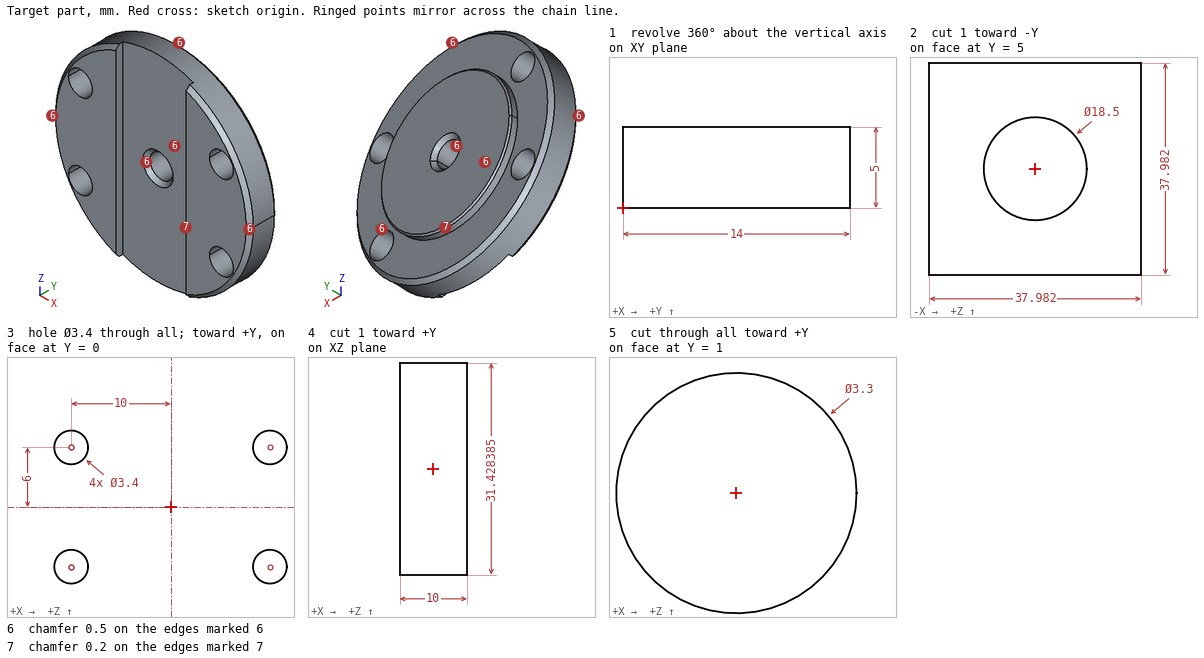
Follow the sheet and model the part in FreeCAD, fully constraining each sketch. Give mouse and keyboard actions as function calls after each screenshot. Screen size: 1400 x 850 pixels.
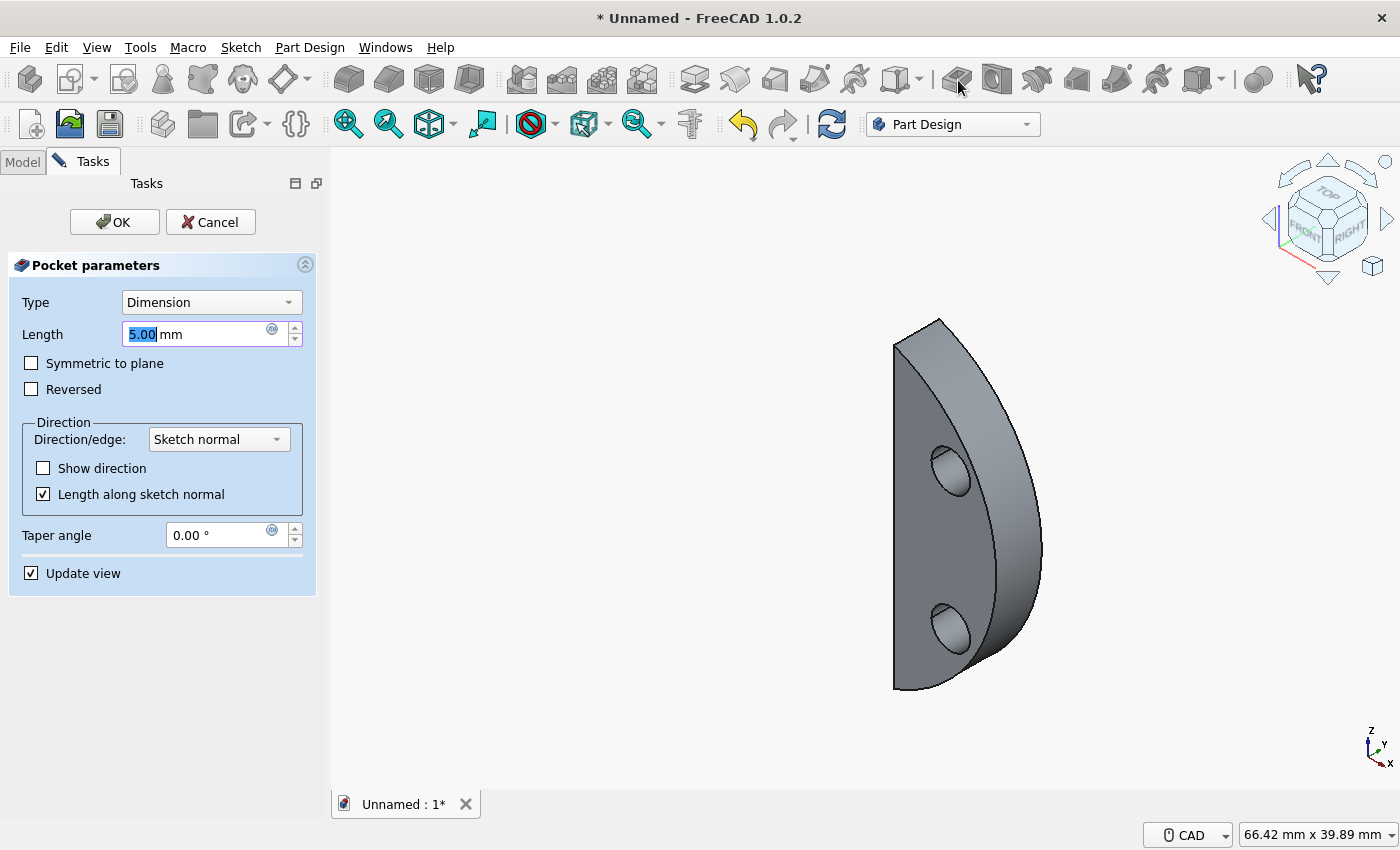
text(1)
key(Tab)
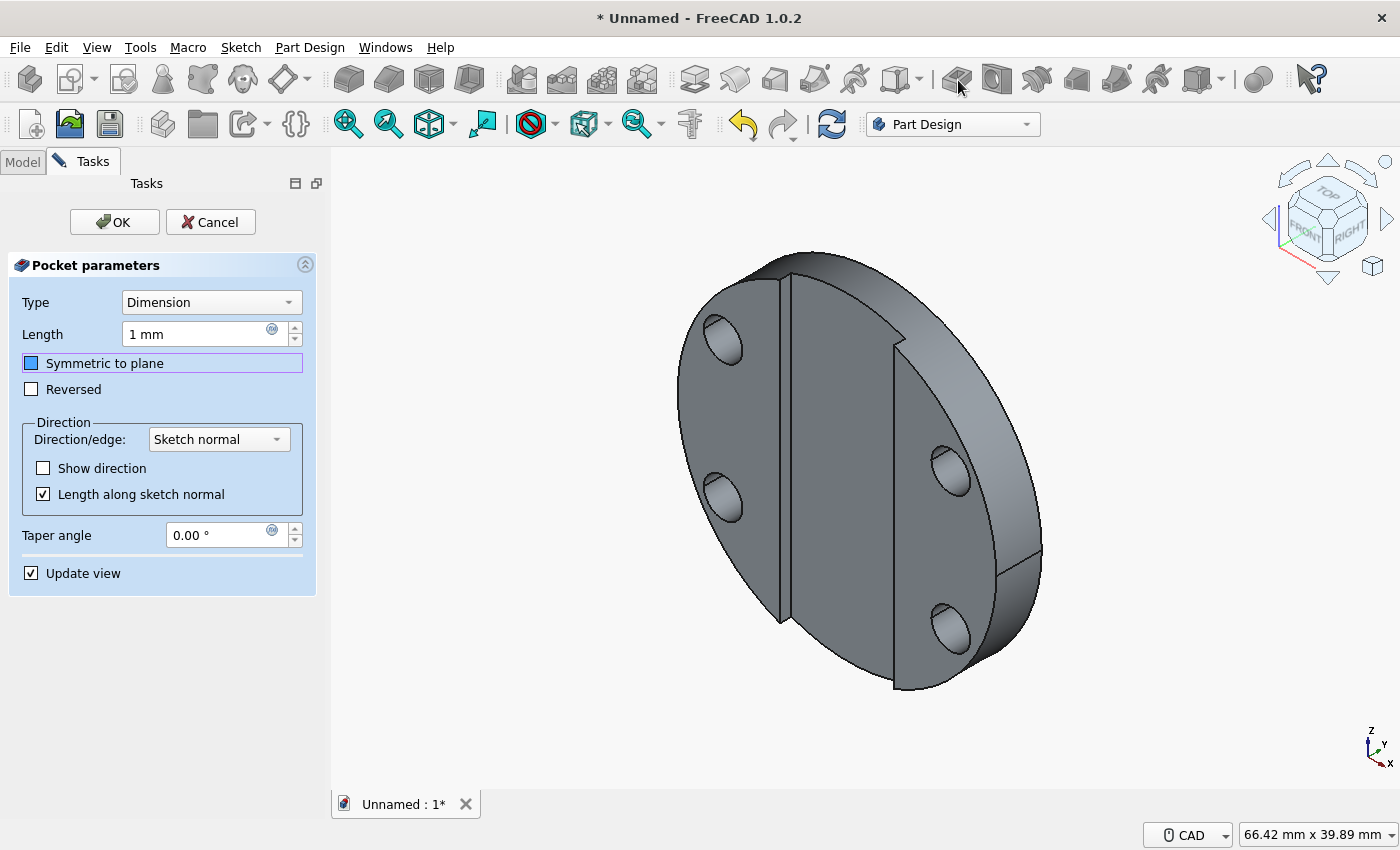
click(115, 222)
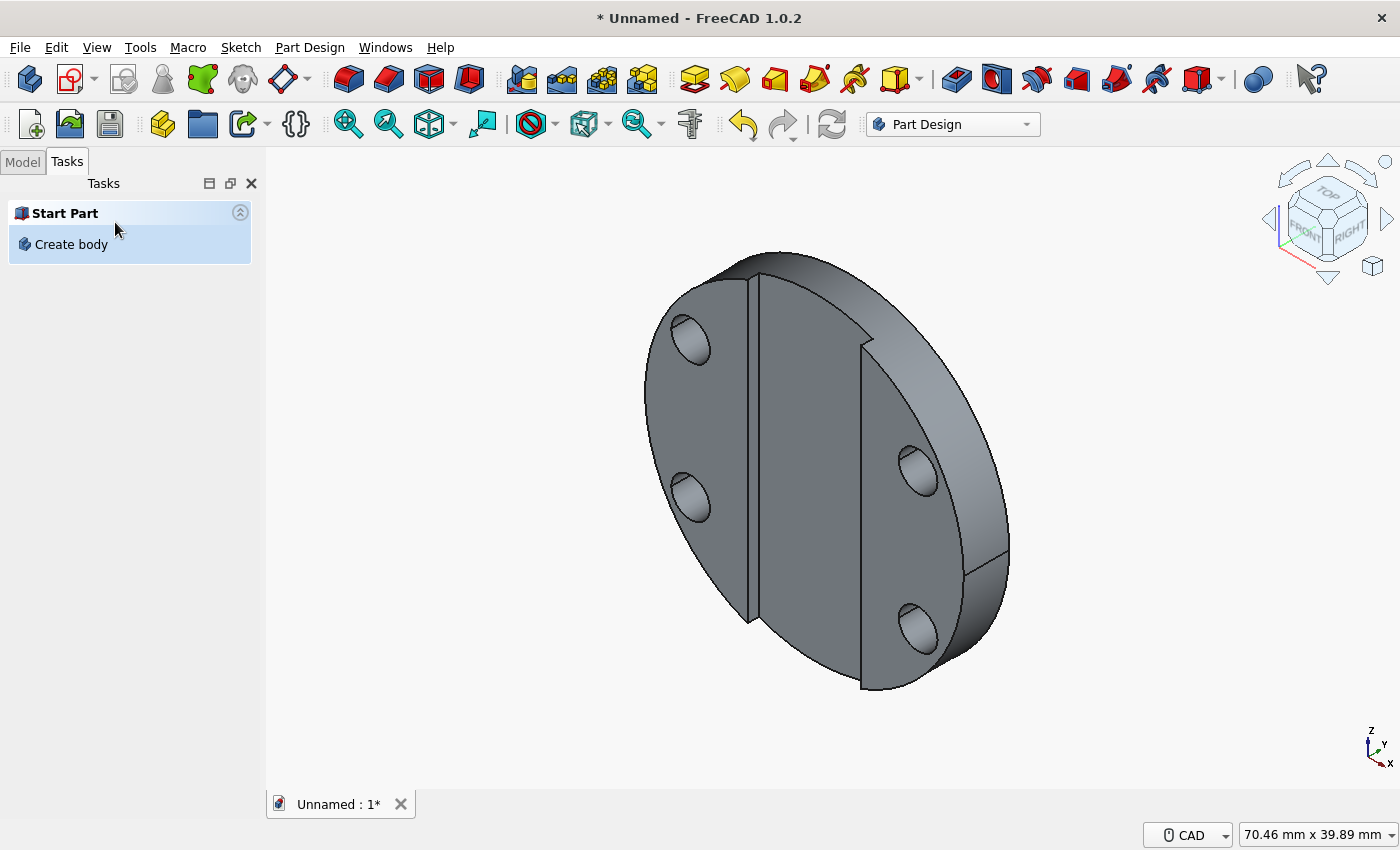
click(816, 372)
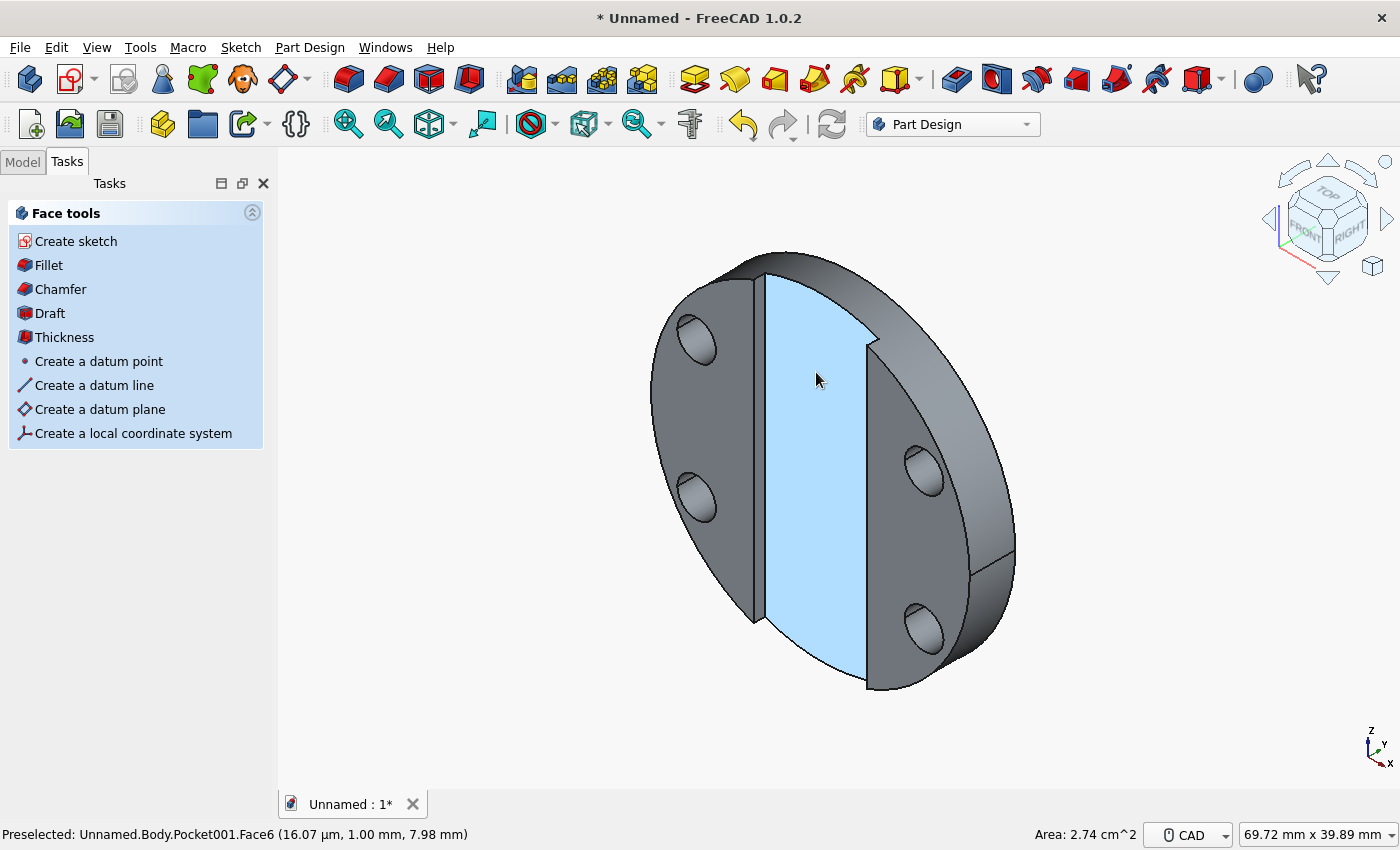
click(70, 80)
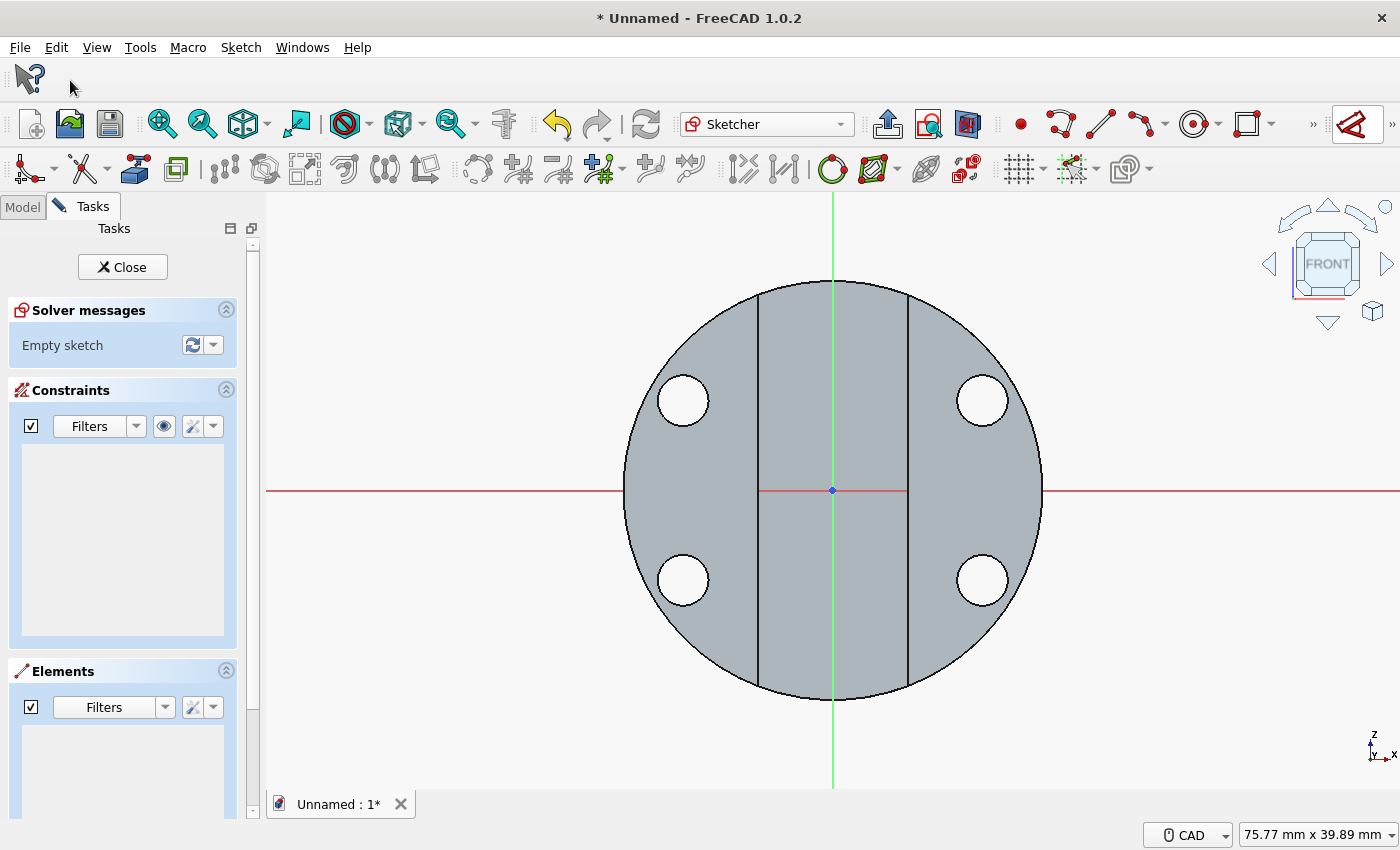
scroll(844, 491, up, 10)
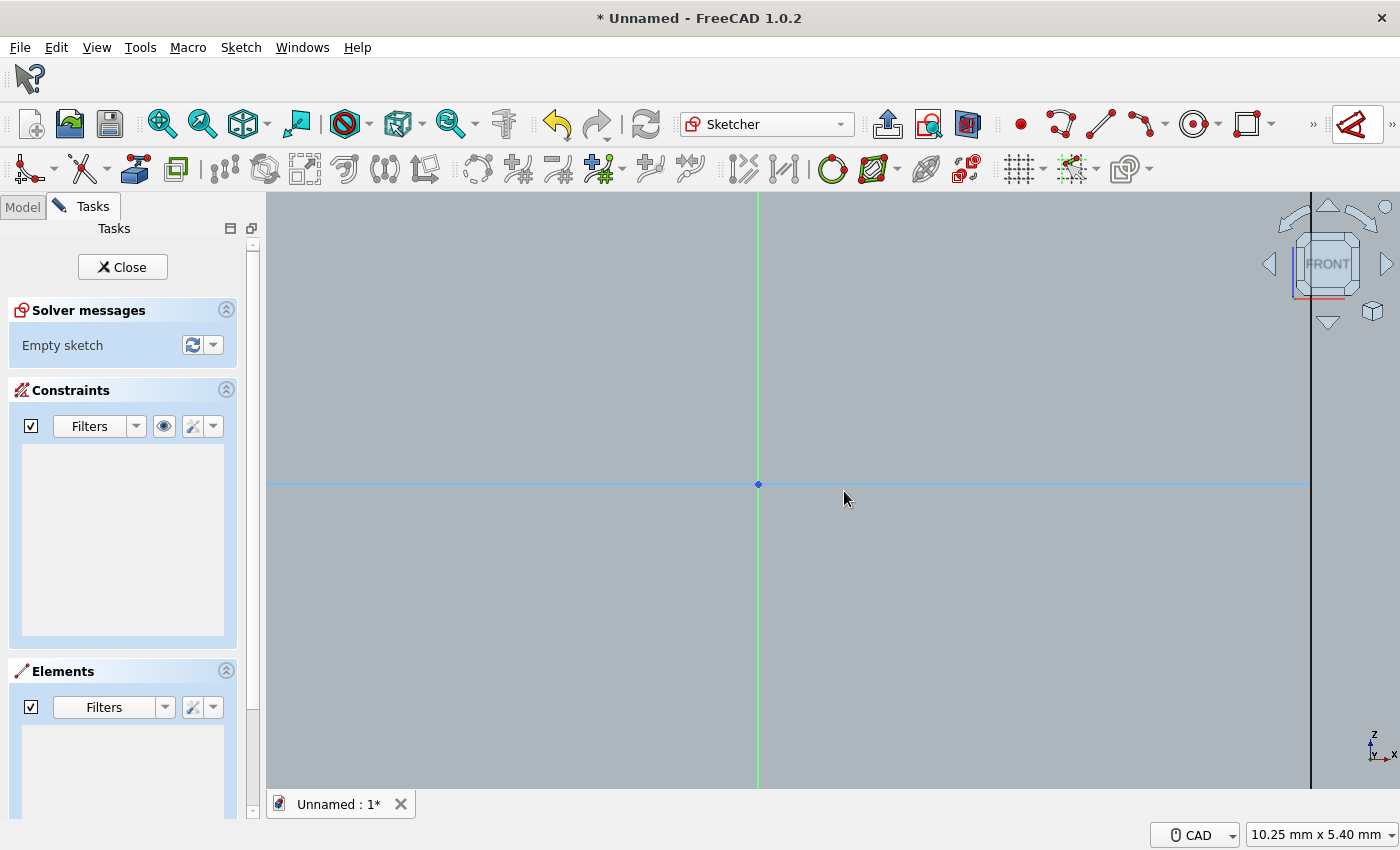
click(1194, 124)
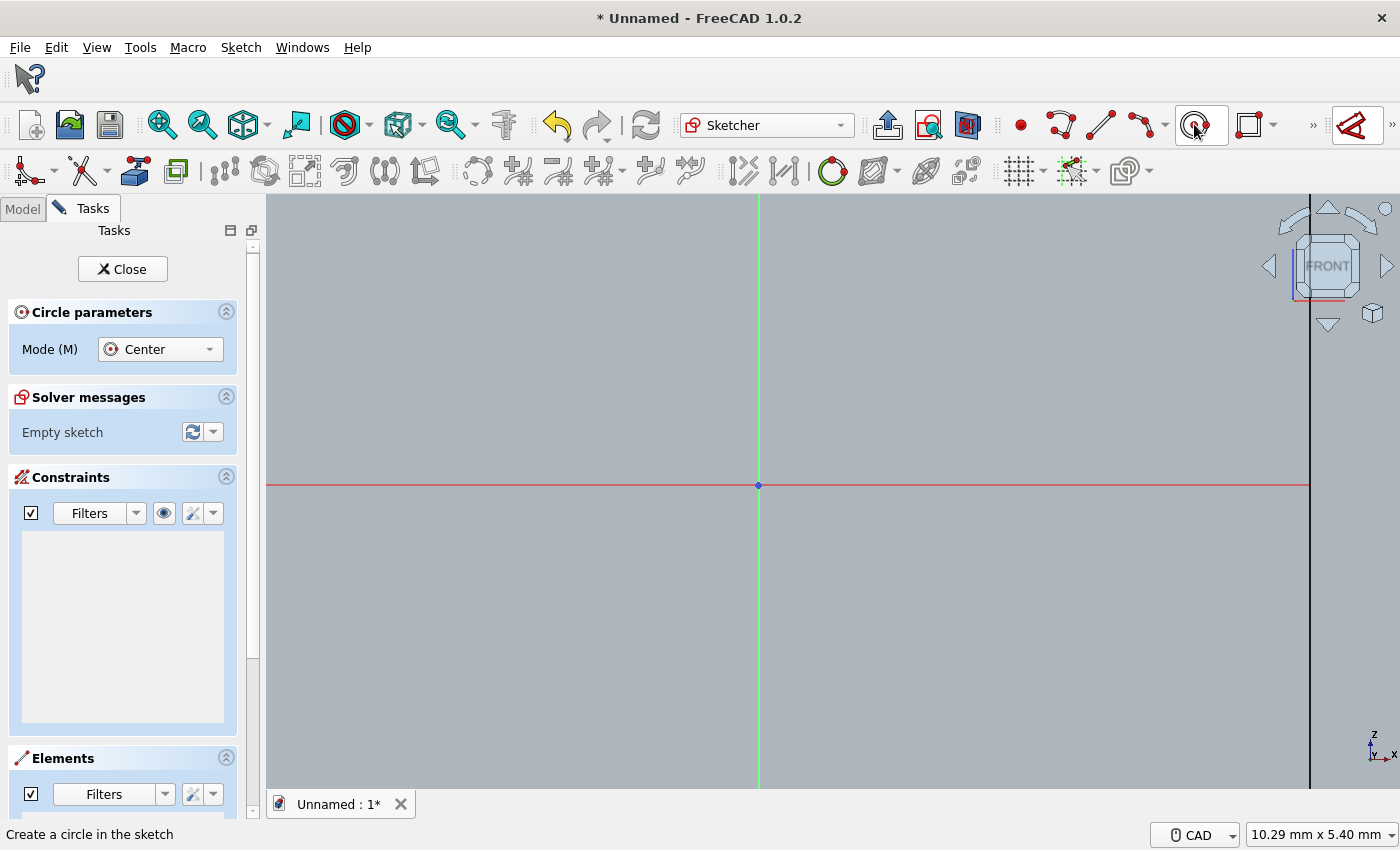
click(759, 485)
move(887, 357)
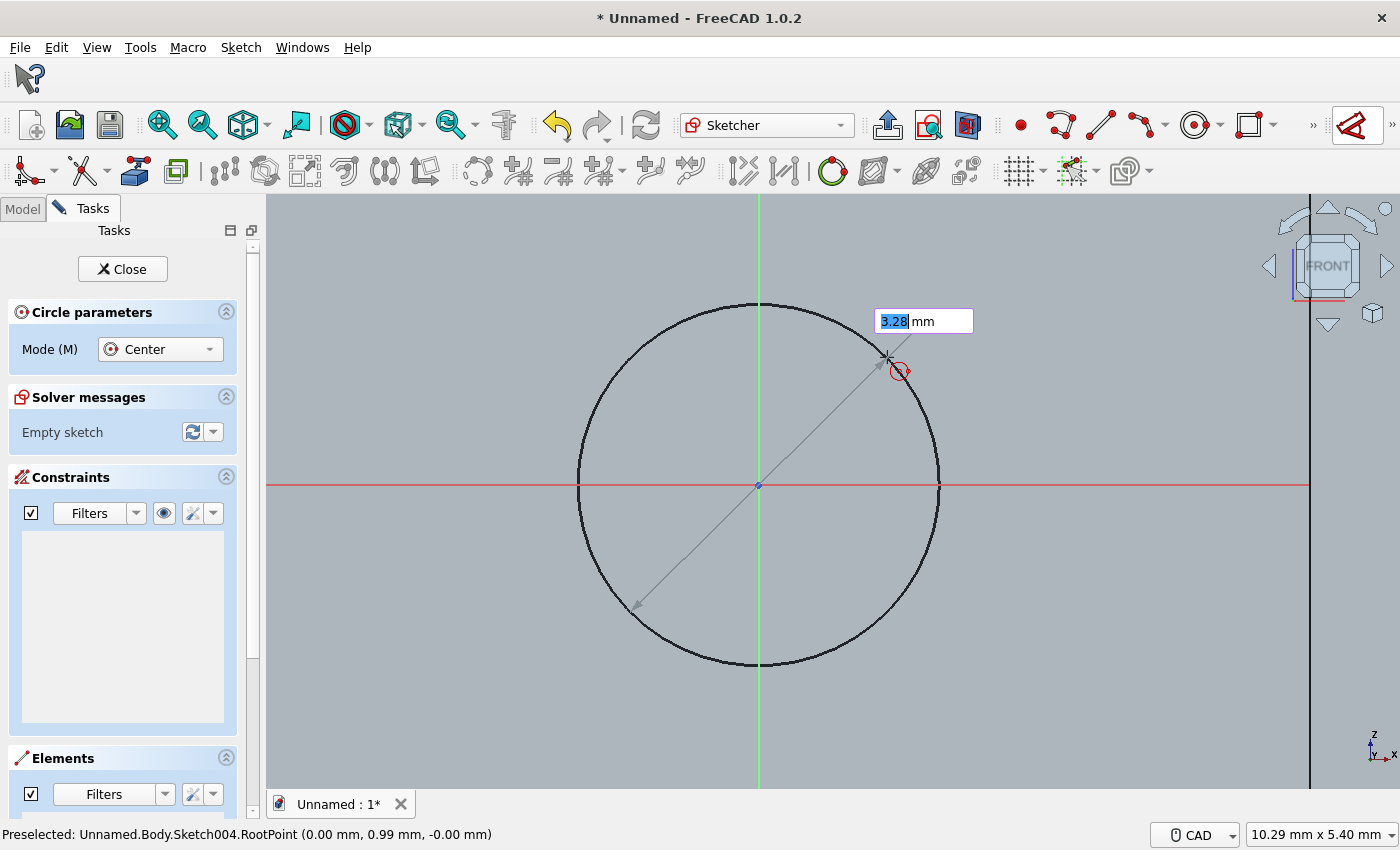
text(3.3)
key(Return)
key(Escape)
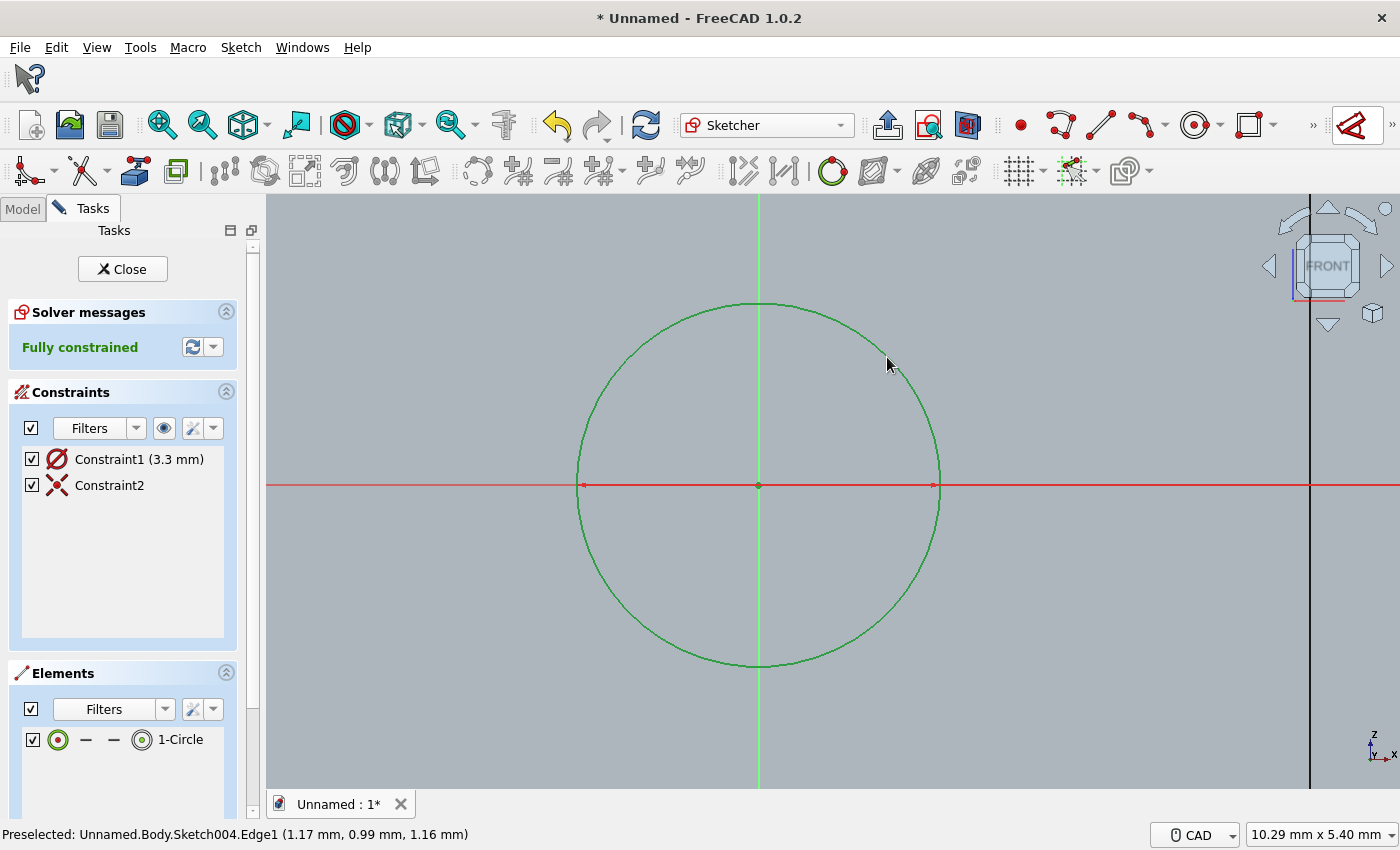
click(123, 269)